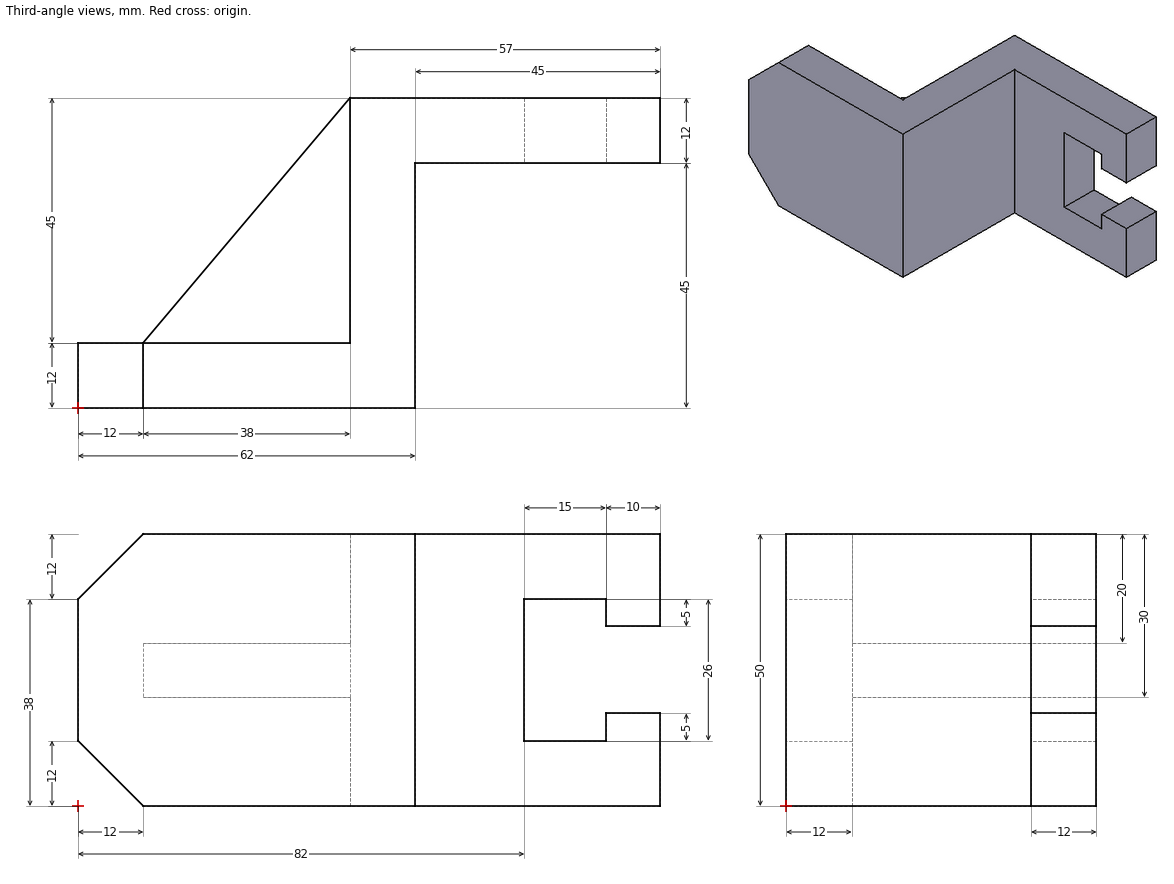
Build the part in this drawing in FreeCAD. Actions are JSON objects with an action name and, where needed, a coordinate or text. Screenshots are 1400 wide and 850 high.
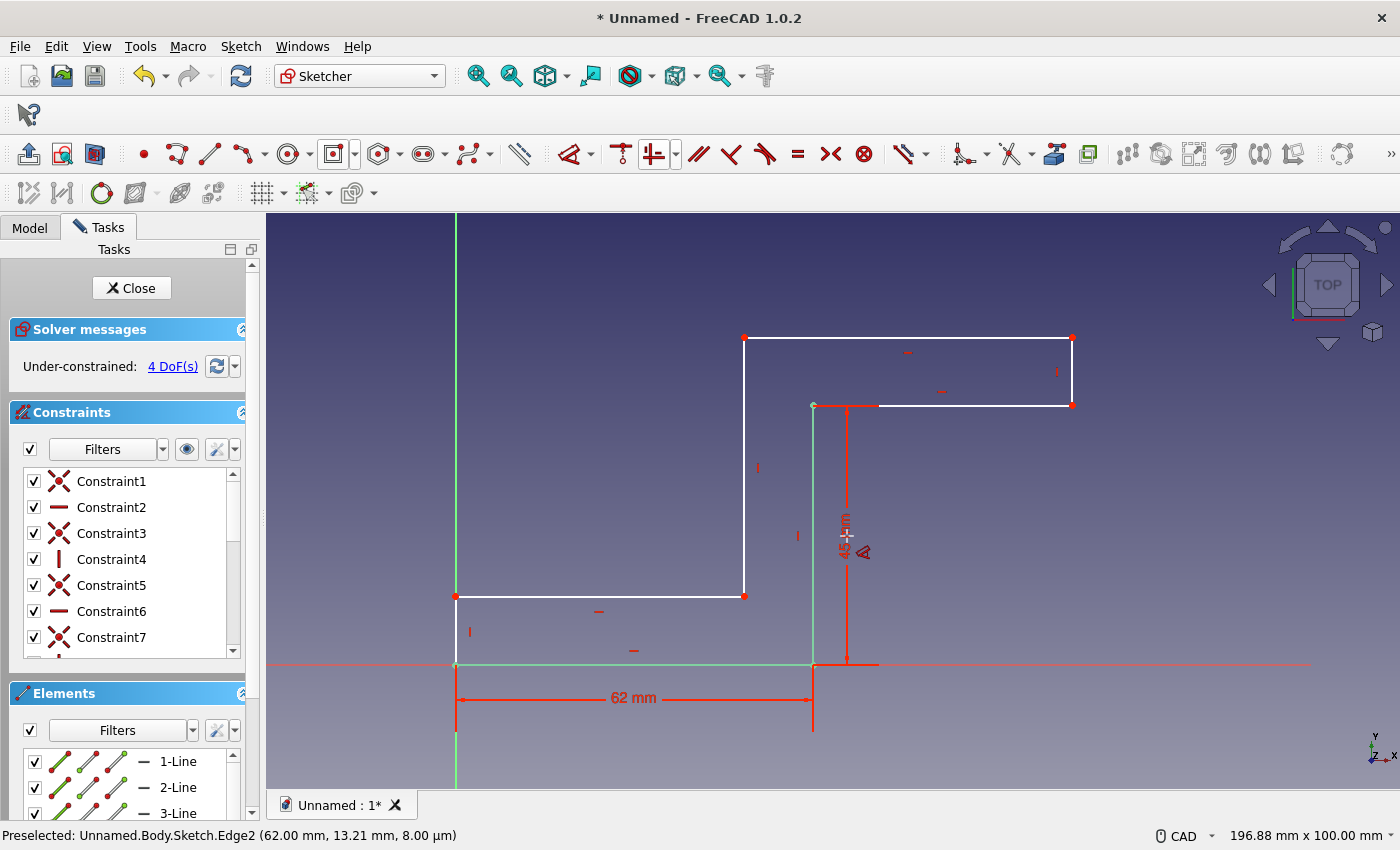
{"action": "left_click", "coordinate": [891, 406]}
{"action": "left_click", "coordinate": [943, 372]}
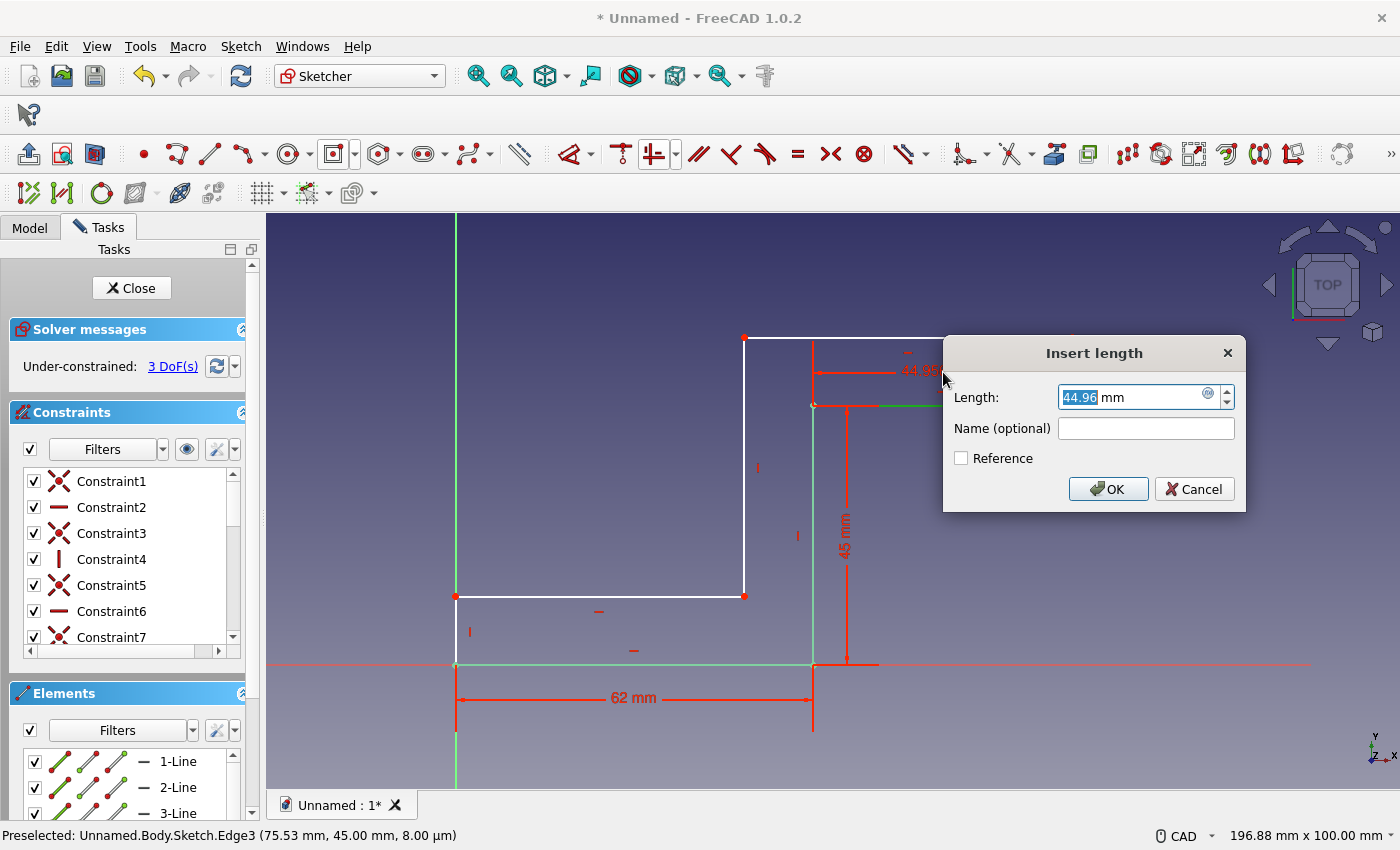
{"action": "type", "text": "45"}
{"action": "key", "text": "Return"}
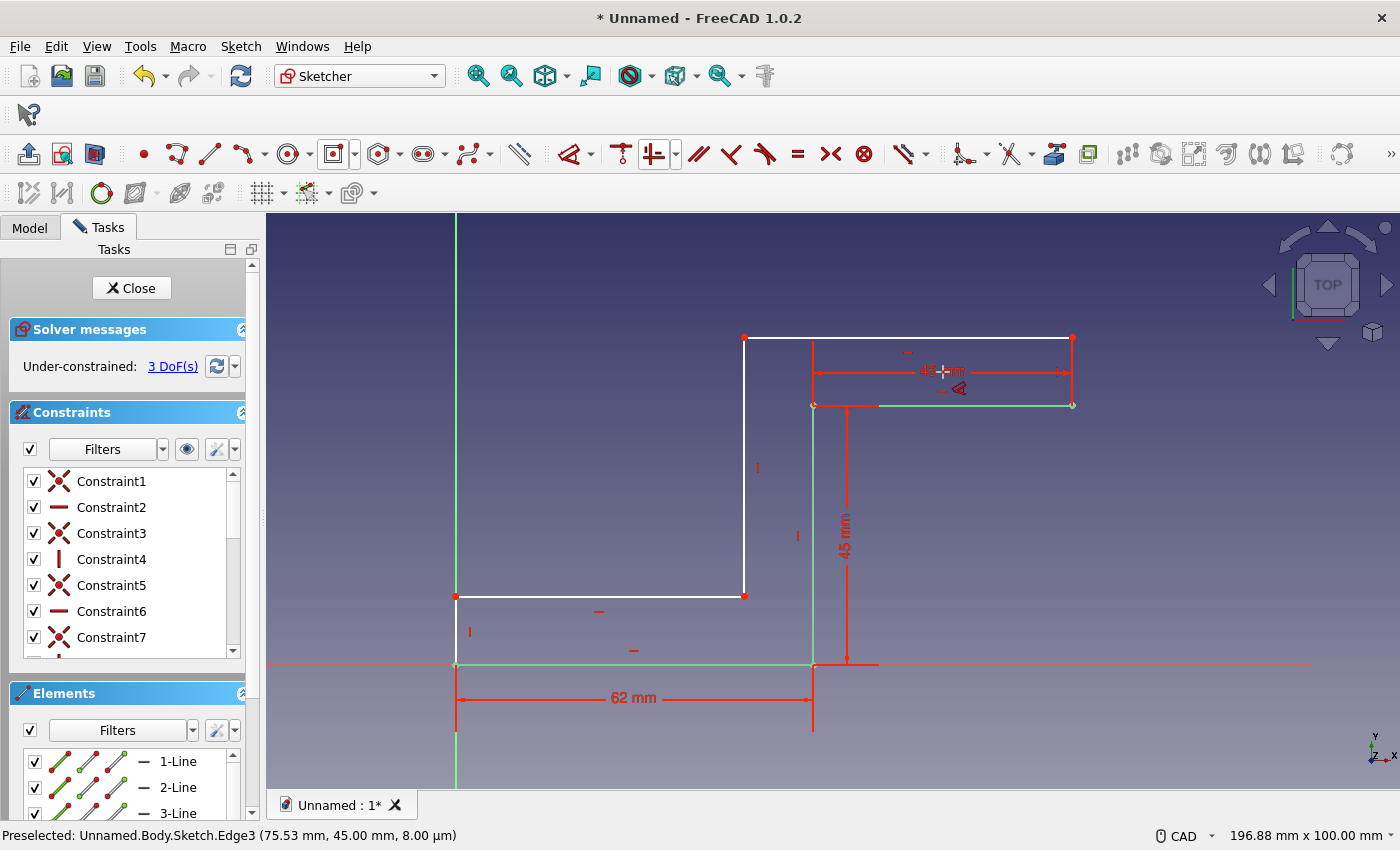
{"action": "left_click", "coordinate": [1072, 386]}
{"action": "left_click", "coordinate": [1106, 372]}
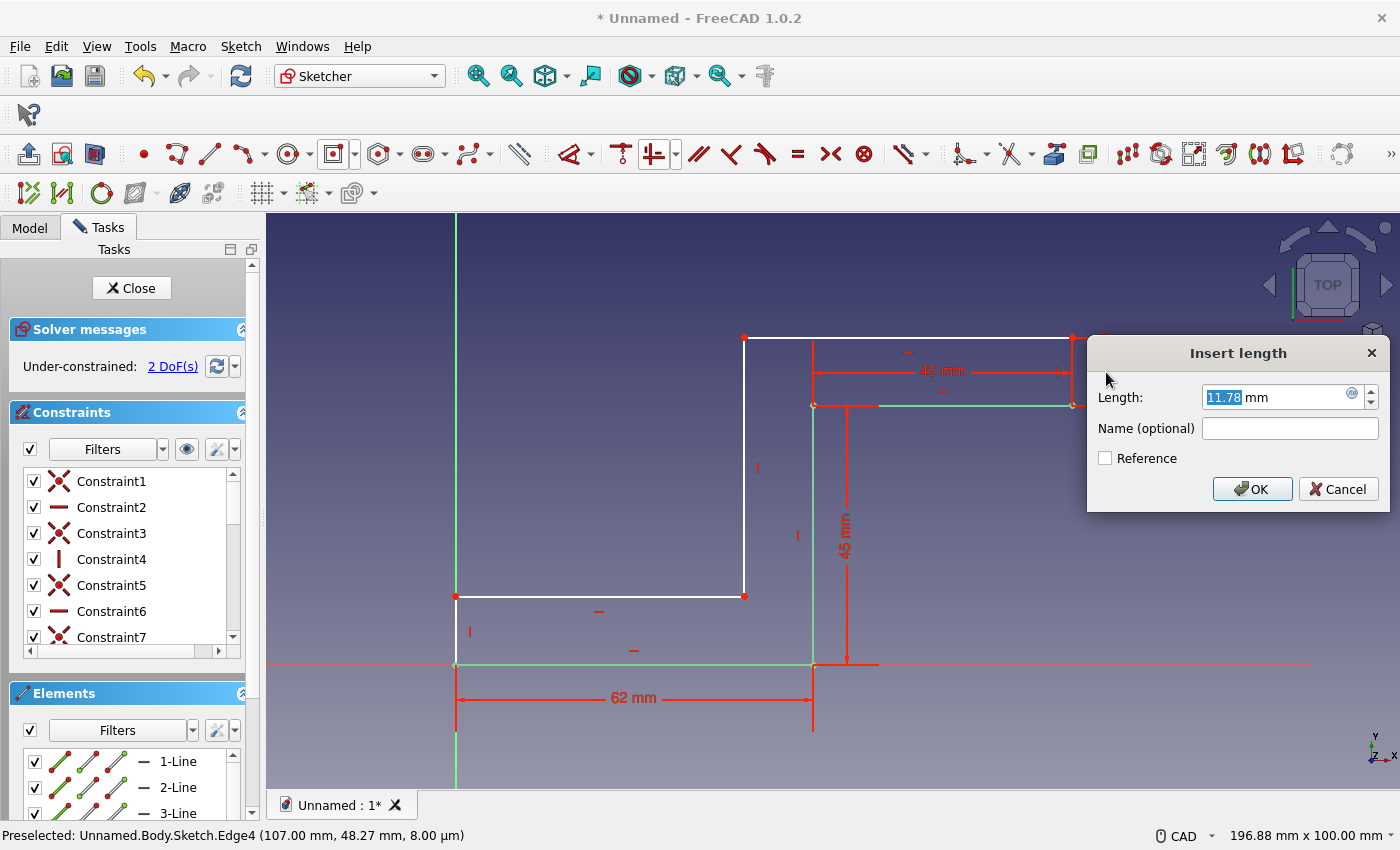
{"action": "type", "text": "12"}
{"action": "key", "text": "Return"}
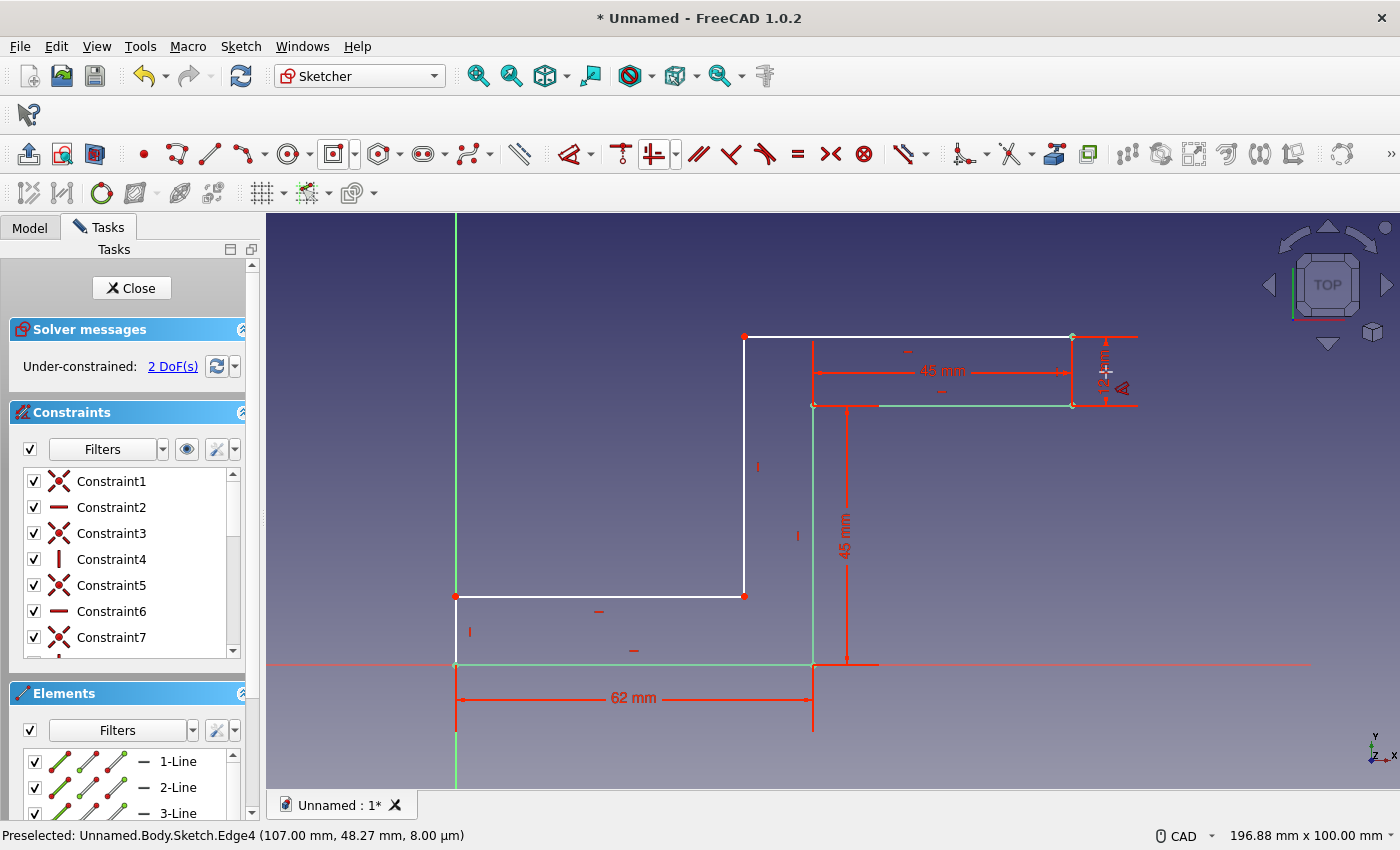
{"action": "left_click", "coordinate": [974, 337]}
{"action": "left_click", "coordinate": [908, 303]}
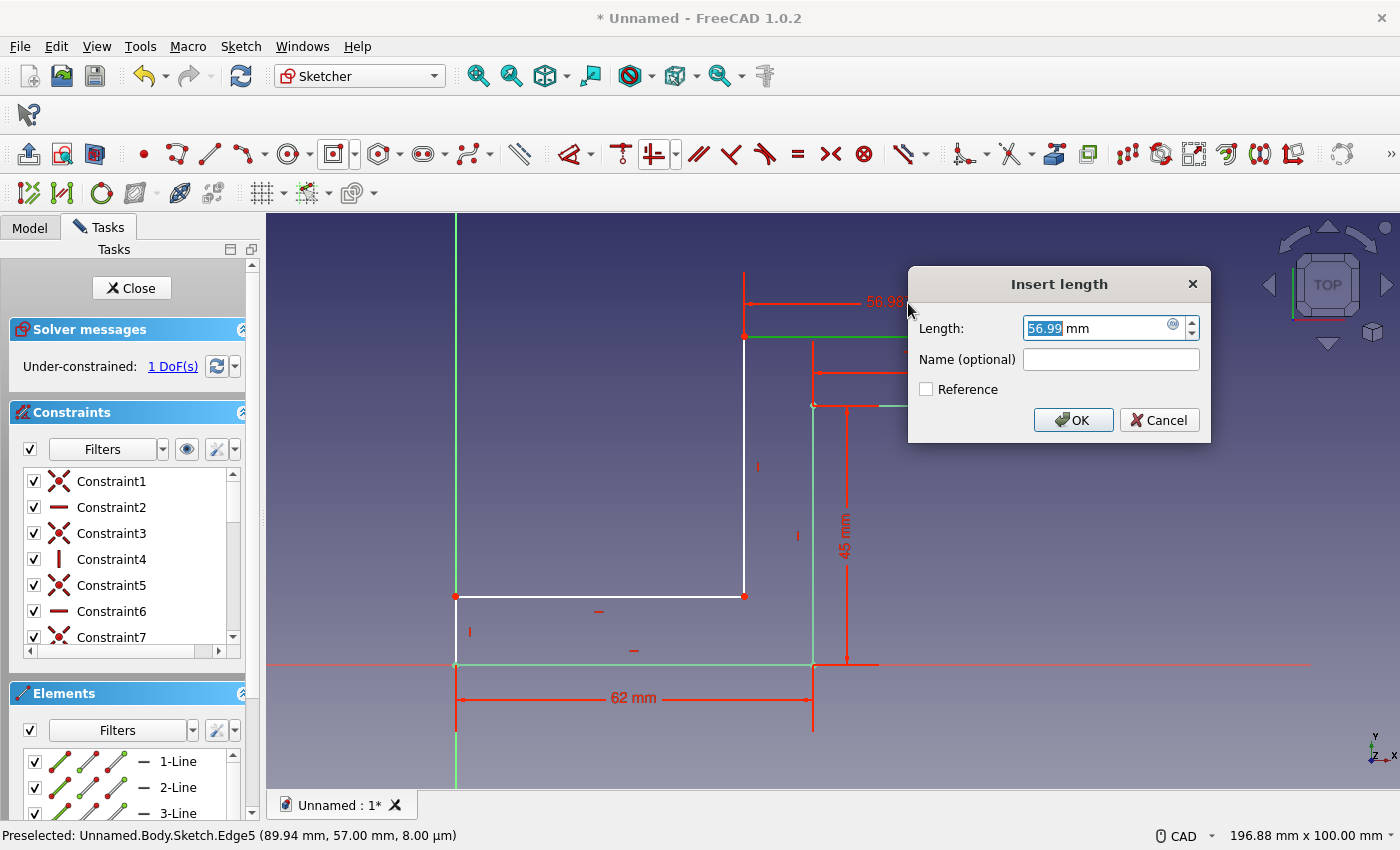
{"action": "type", "text": "57"}
{"action": "key", "text": "Return"}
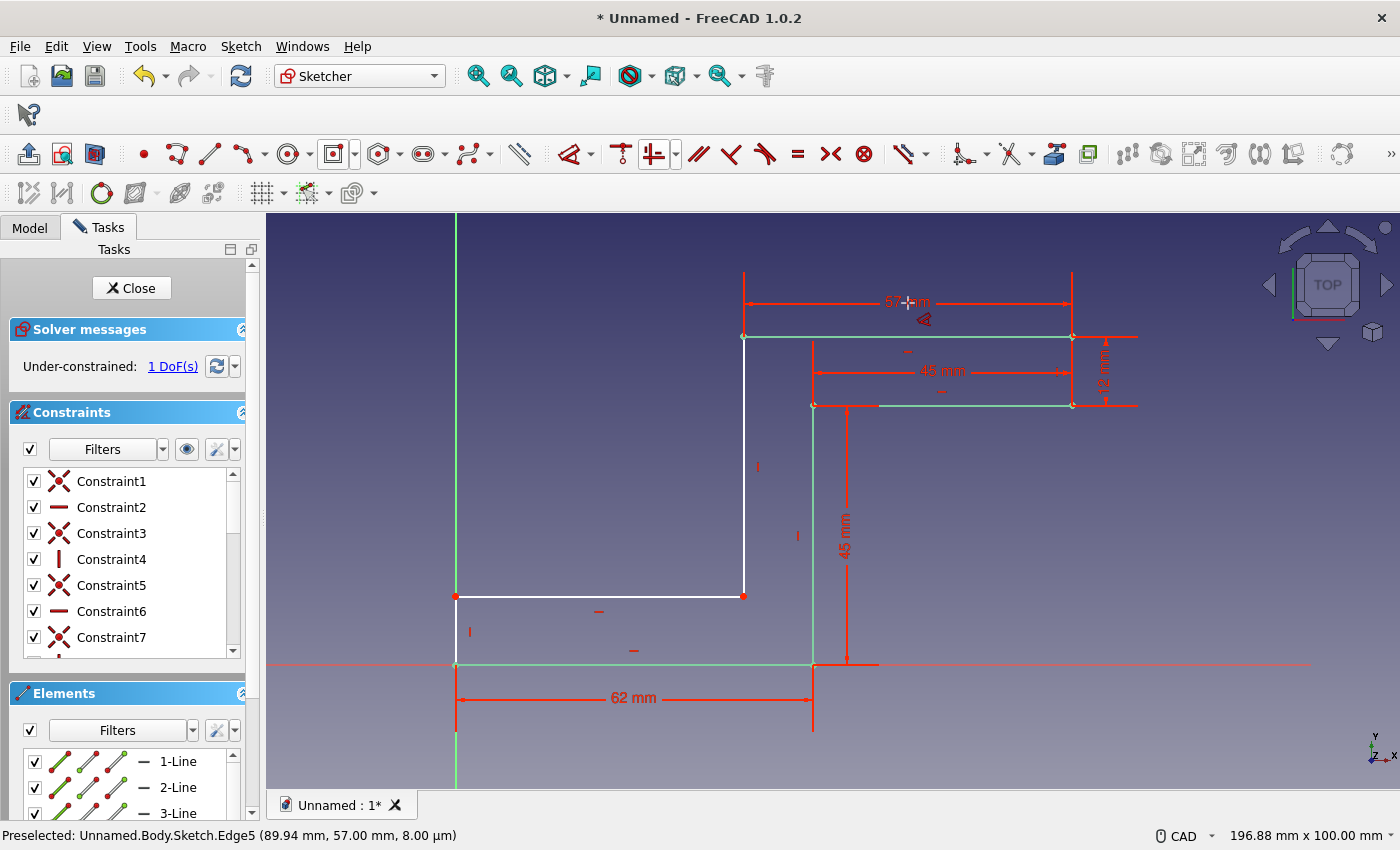
{"action": "left_click", "coordinate": [744, 415]}
{"action": "left_click", "coordinate": [710, 467]}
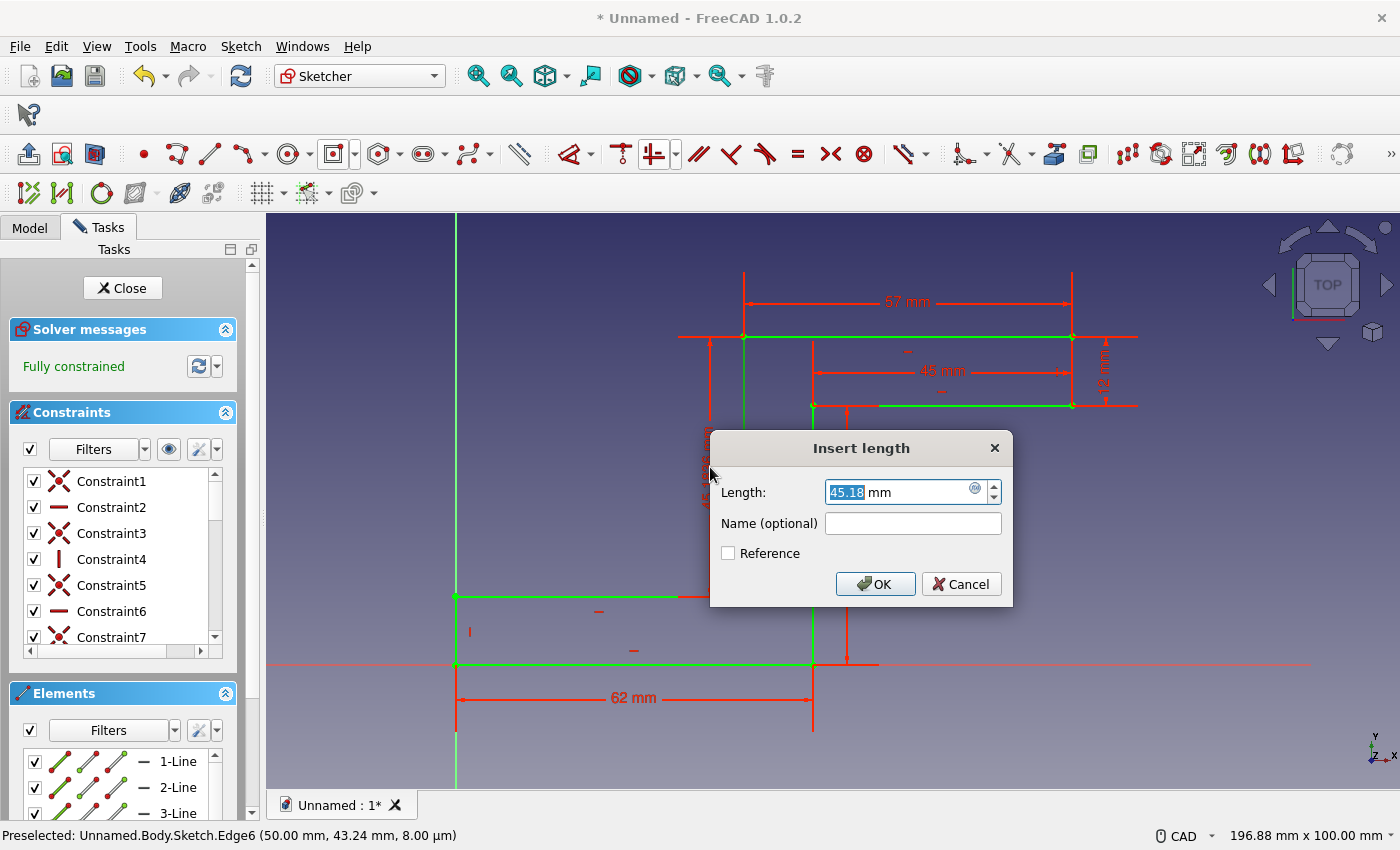
{"action": "type", "text": "45"}
{"action": "key", "text": "Return"}
{"action": "key", "text": "Escape"}